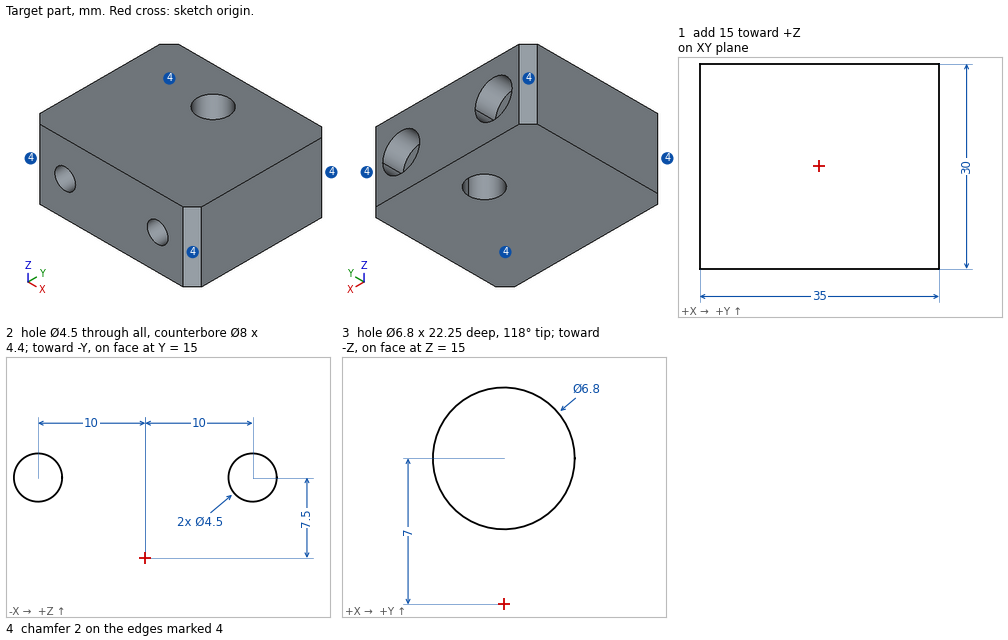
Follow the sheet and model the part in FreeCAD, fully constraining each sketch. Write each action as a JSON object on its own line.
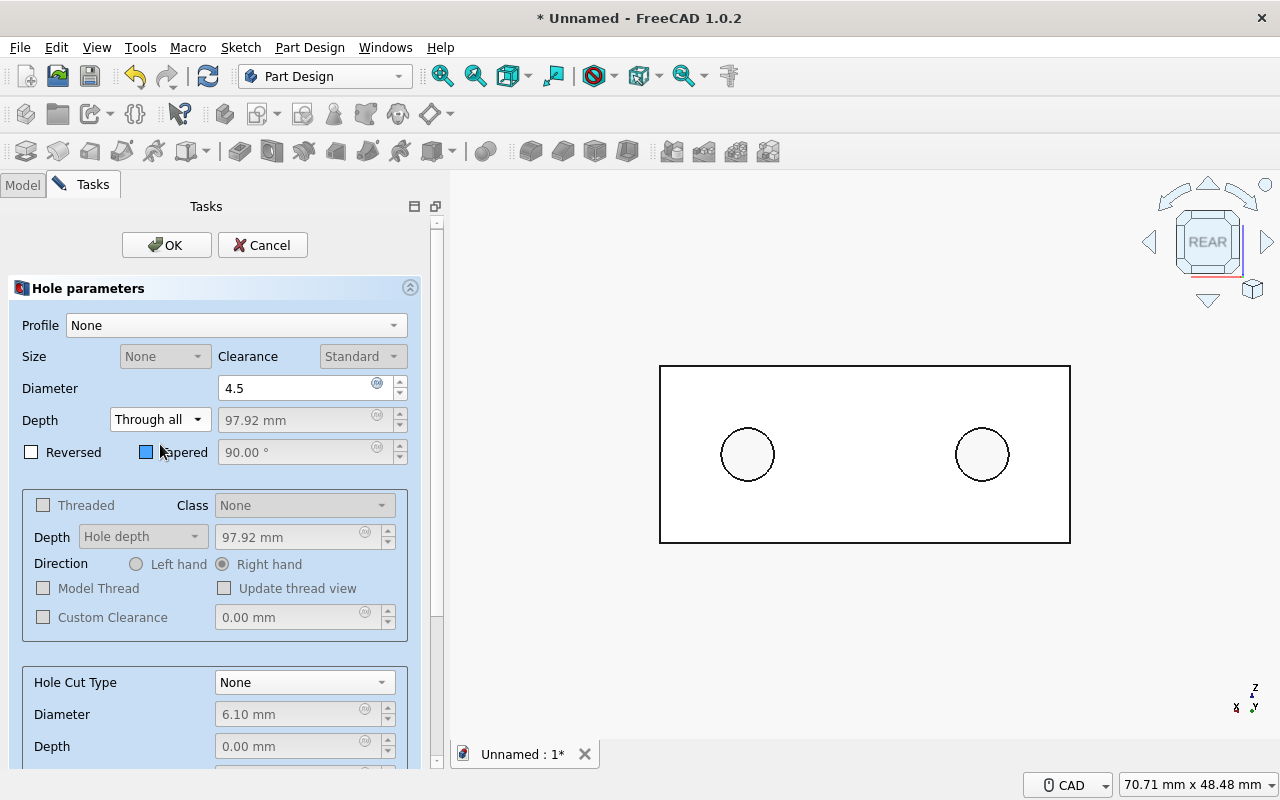
{"action": "left_click", "coordinate": [306, 682]}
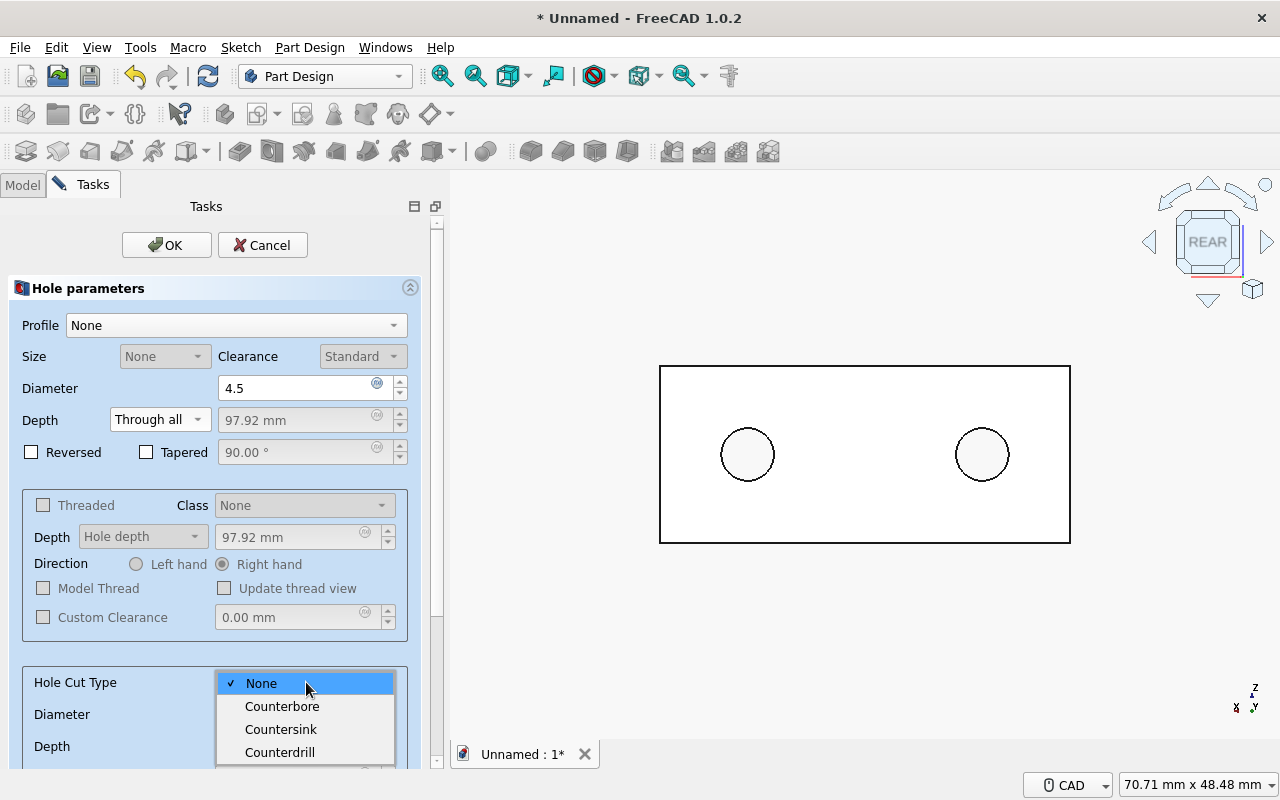
{"action": "left_click", "coordinate": [304, 706]}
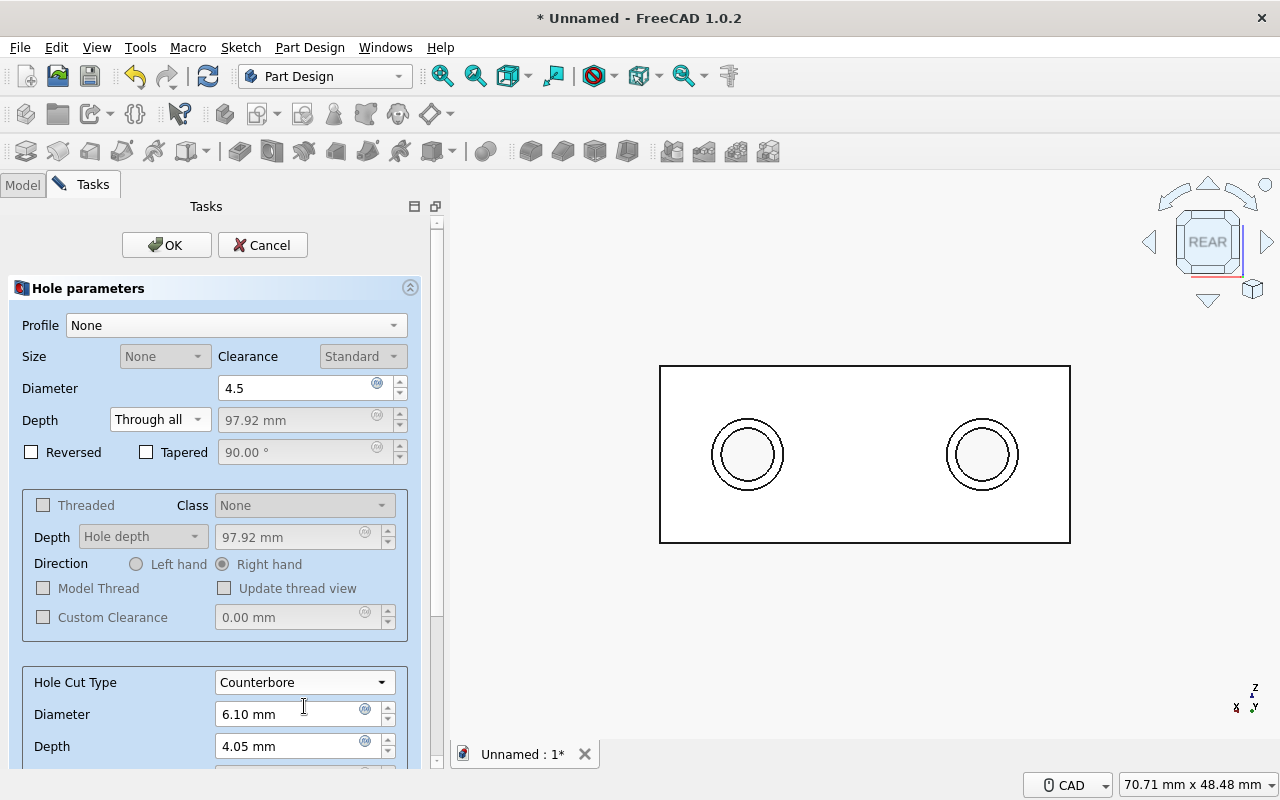
{"action": "triple_click", "coordinate": [298, 714]}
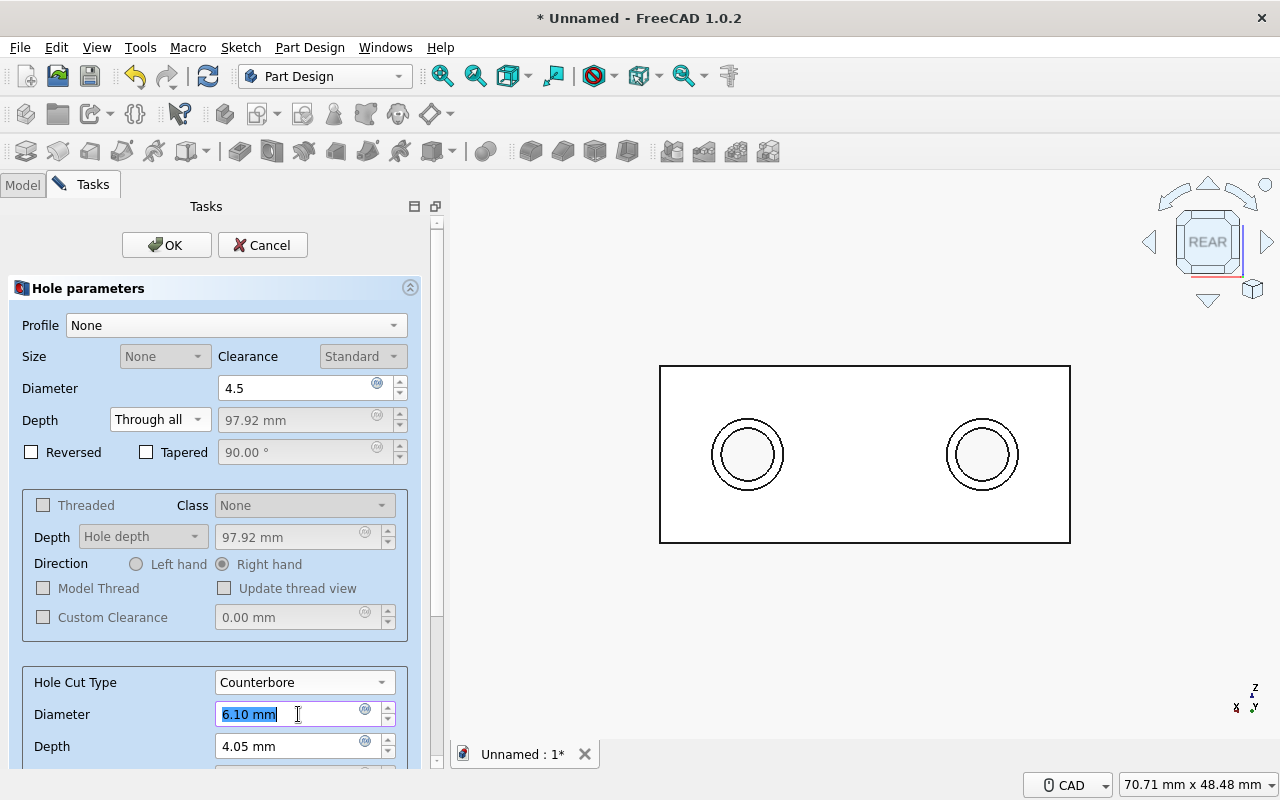
{"action": "type", "text": "8"}
{"action": "key", "text": "Tab"}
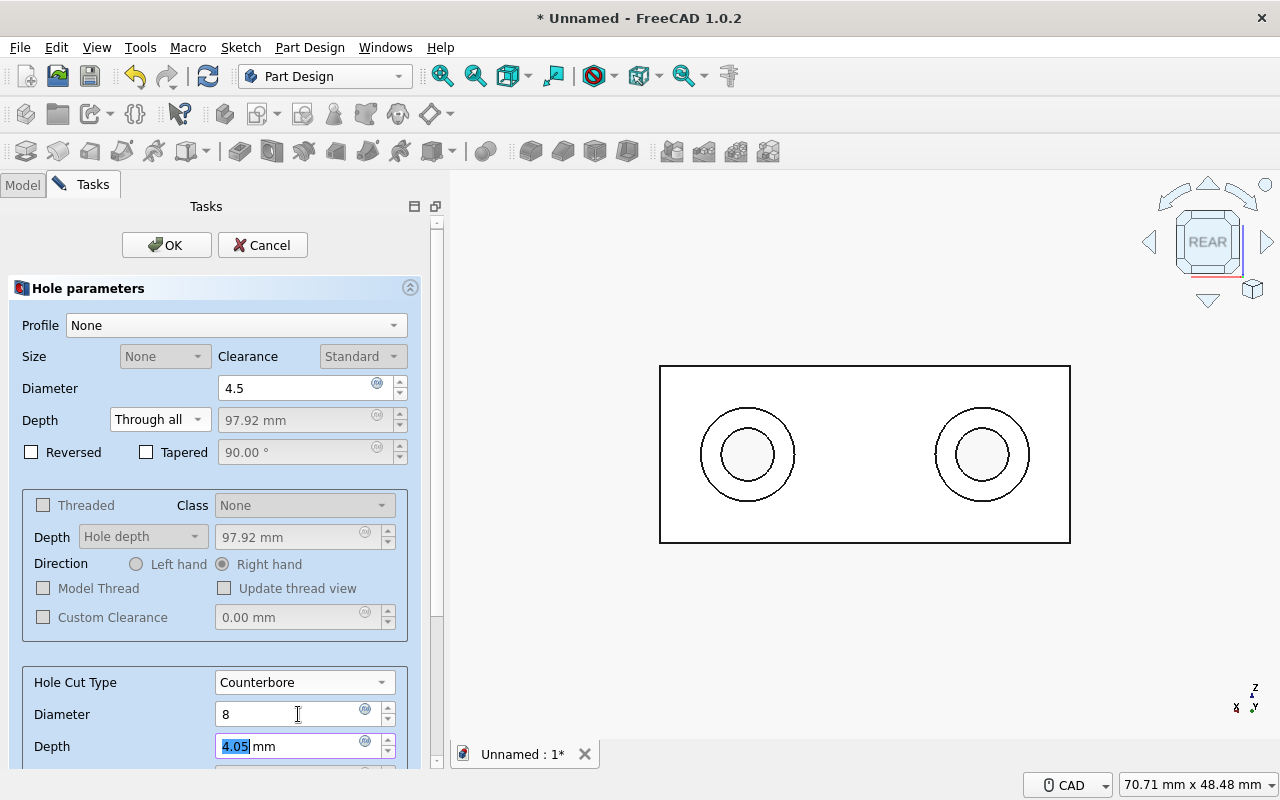
{"action": "type", "text": "4.4"}
{"action": "key", "text": "Tab"}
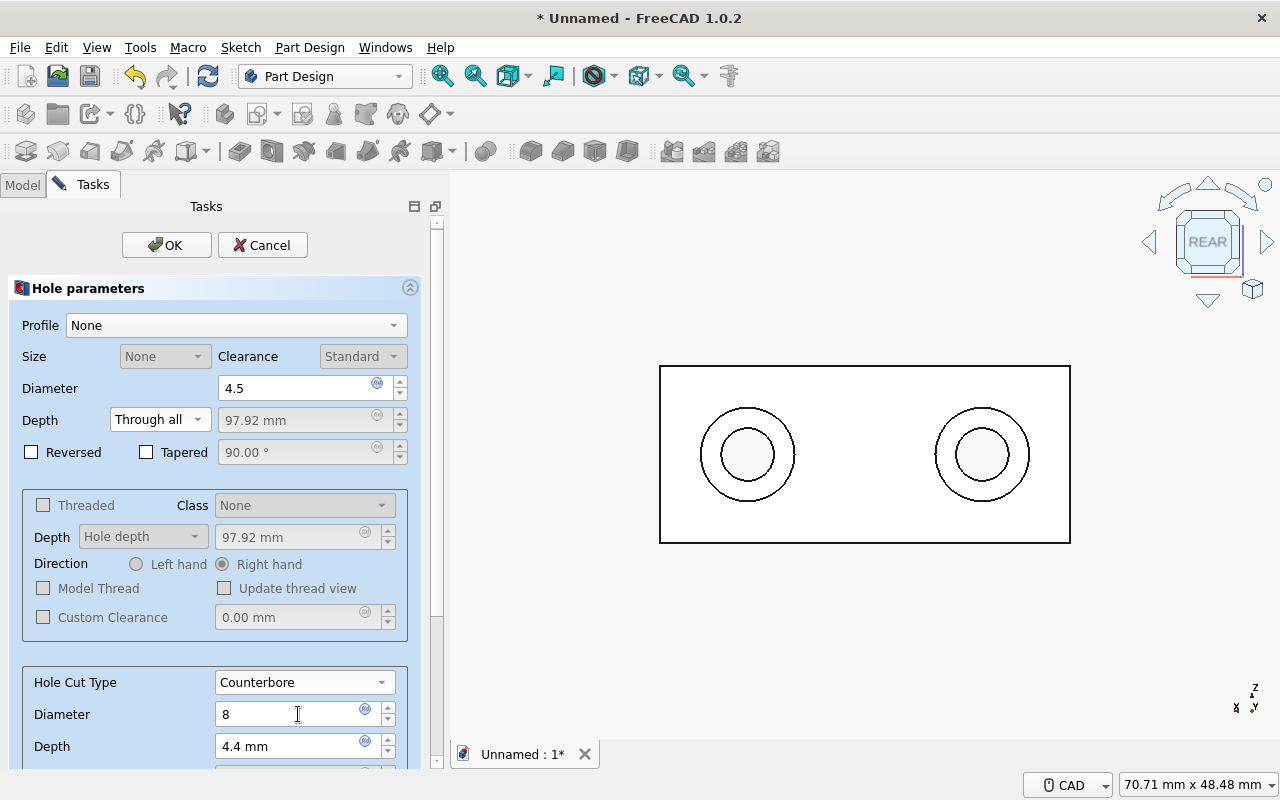
{"action": "left_click", "coordinate": [167, 245]}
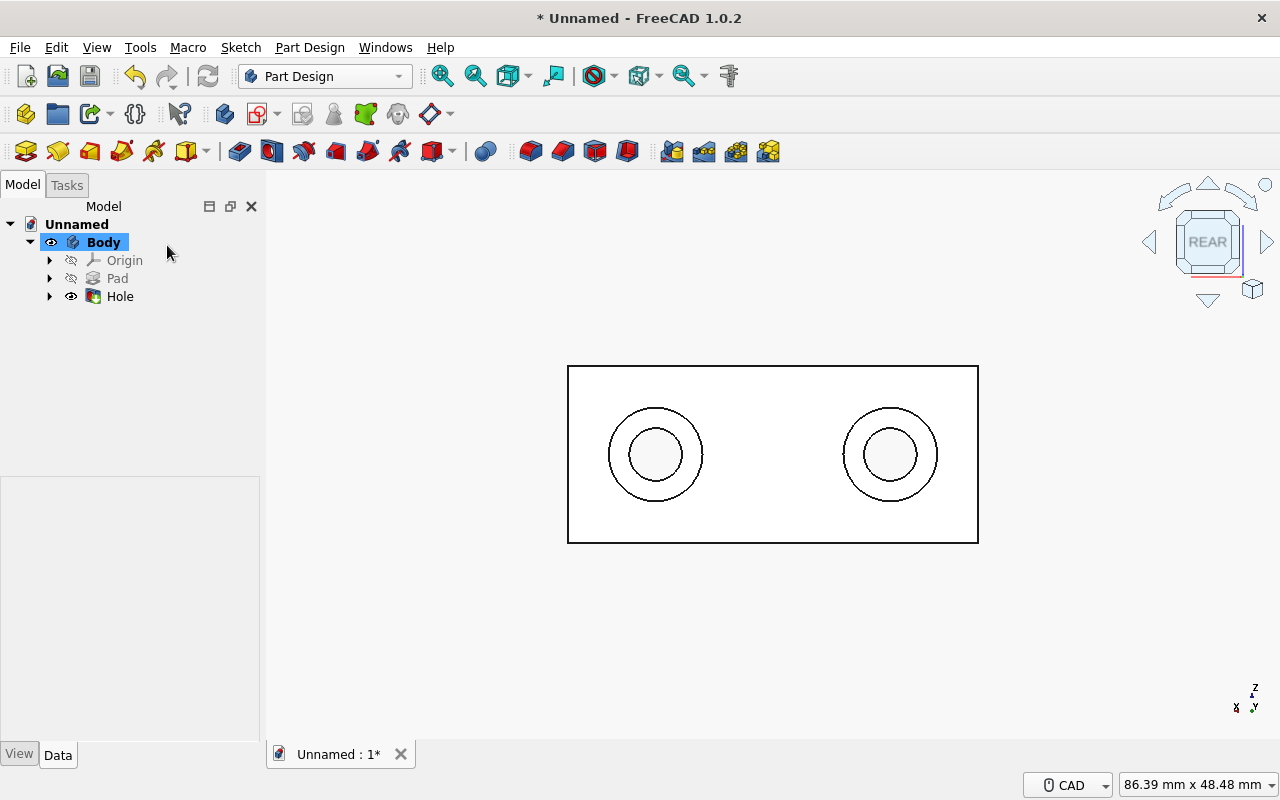
{"action": "key", "text": "v f"}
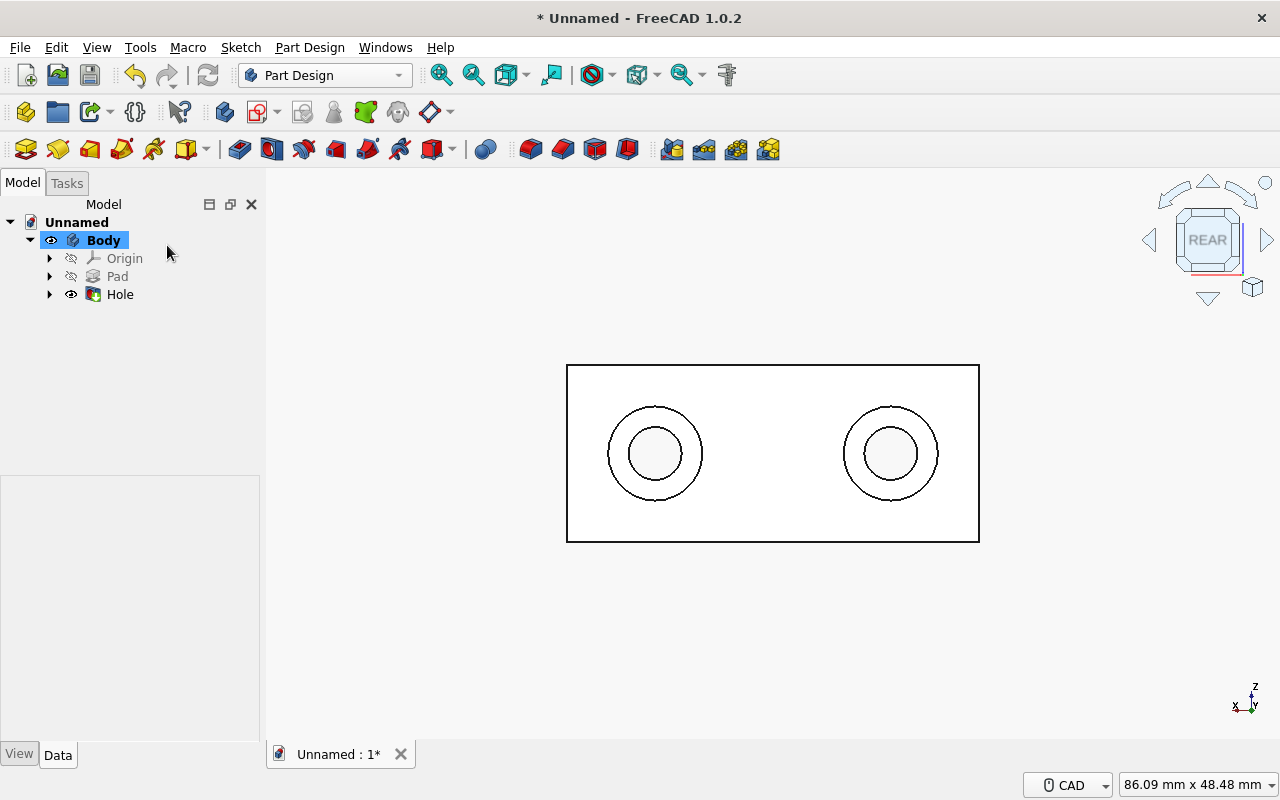
{"action": "key", "text": "0"}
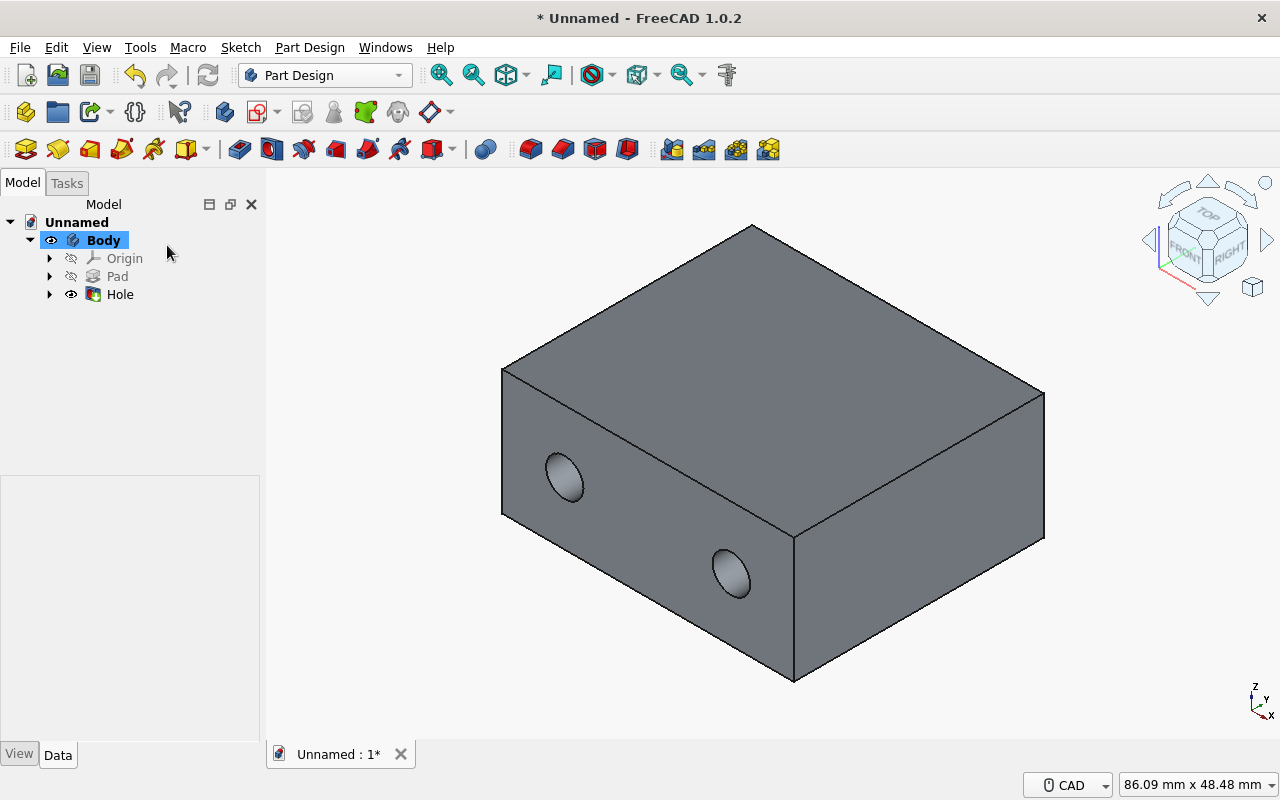
{"action": "left_click", "coordinate": [773, 380]}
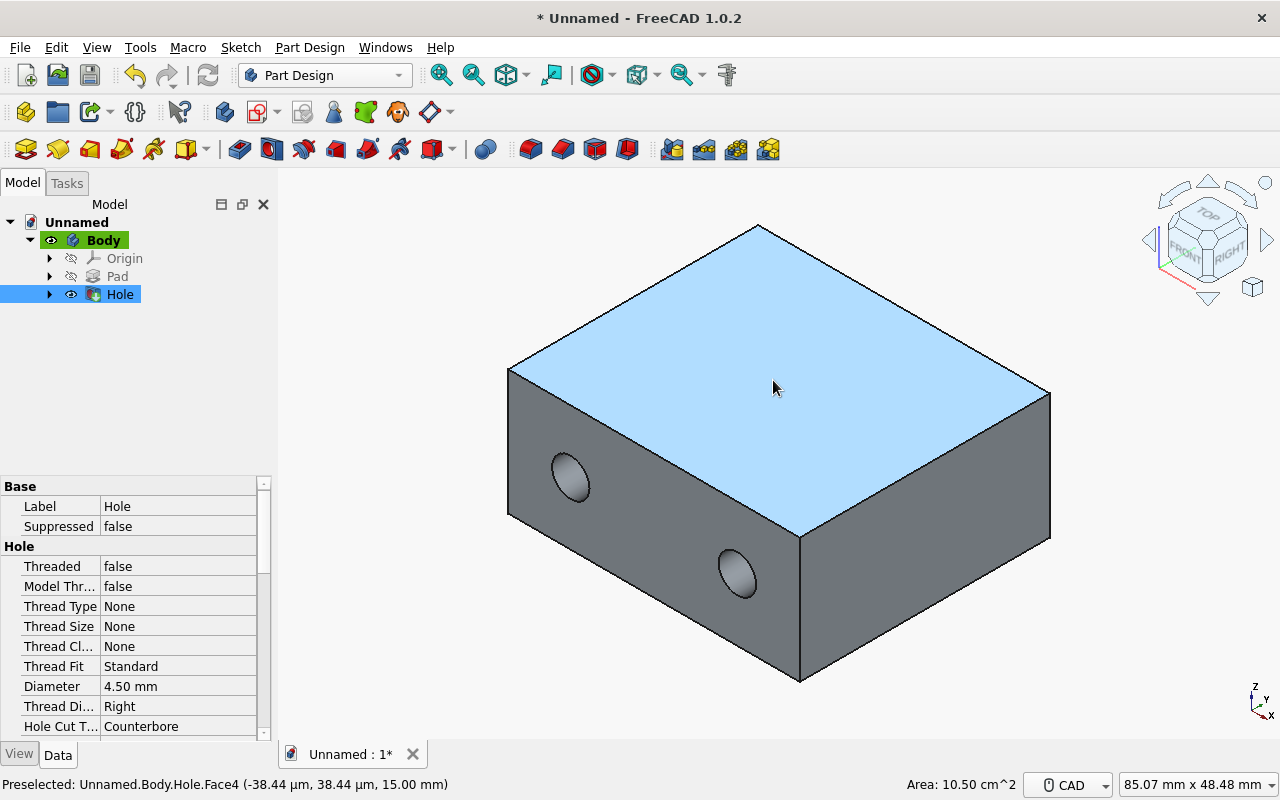
{"action": "left_click", "coordinate": [258, 112]}